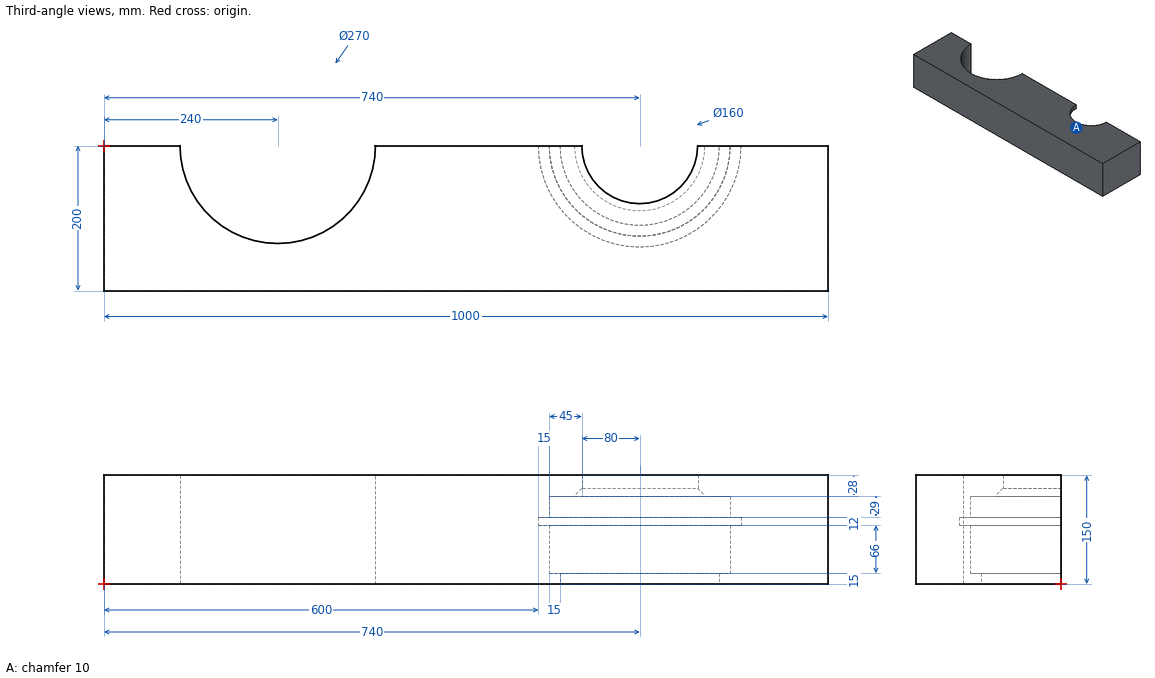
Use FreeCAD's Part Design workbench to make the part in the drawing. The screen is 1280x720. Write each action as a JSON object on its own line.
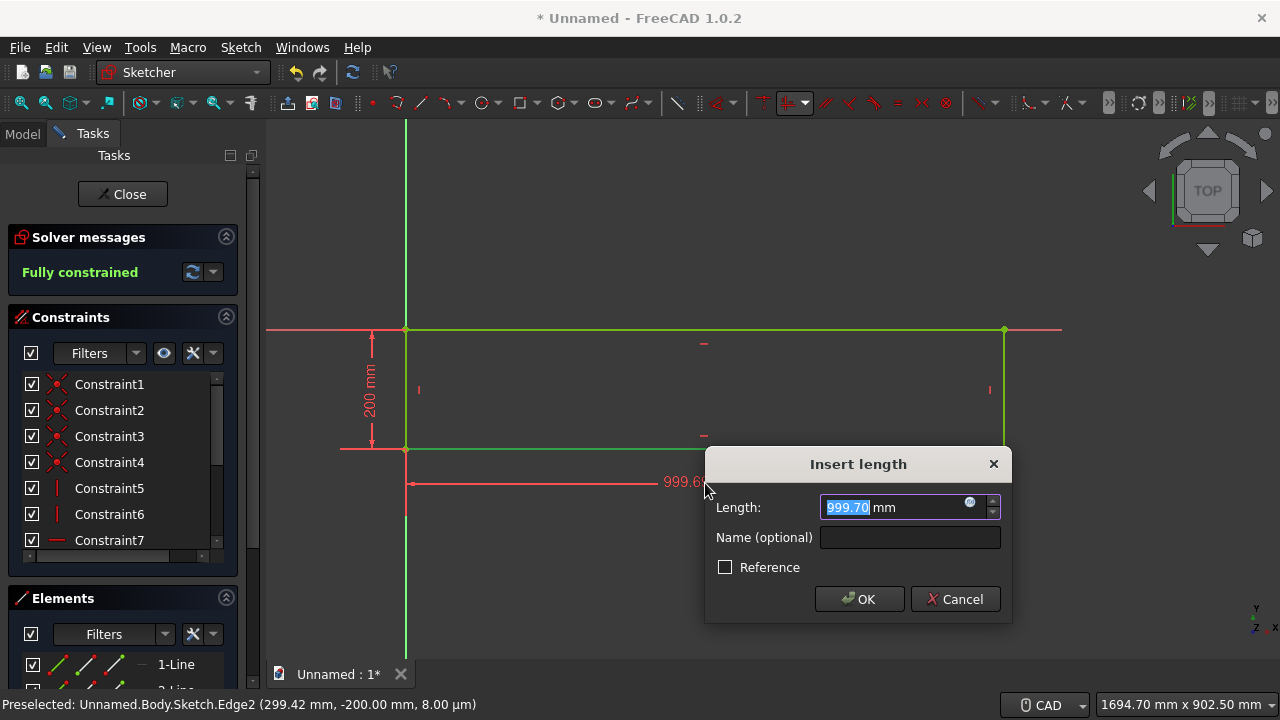
{"action": "type", "text": "1000"}
{"action": "key", "text": "Return"}
{"action": "key", "text": "Escape"}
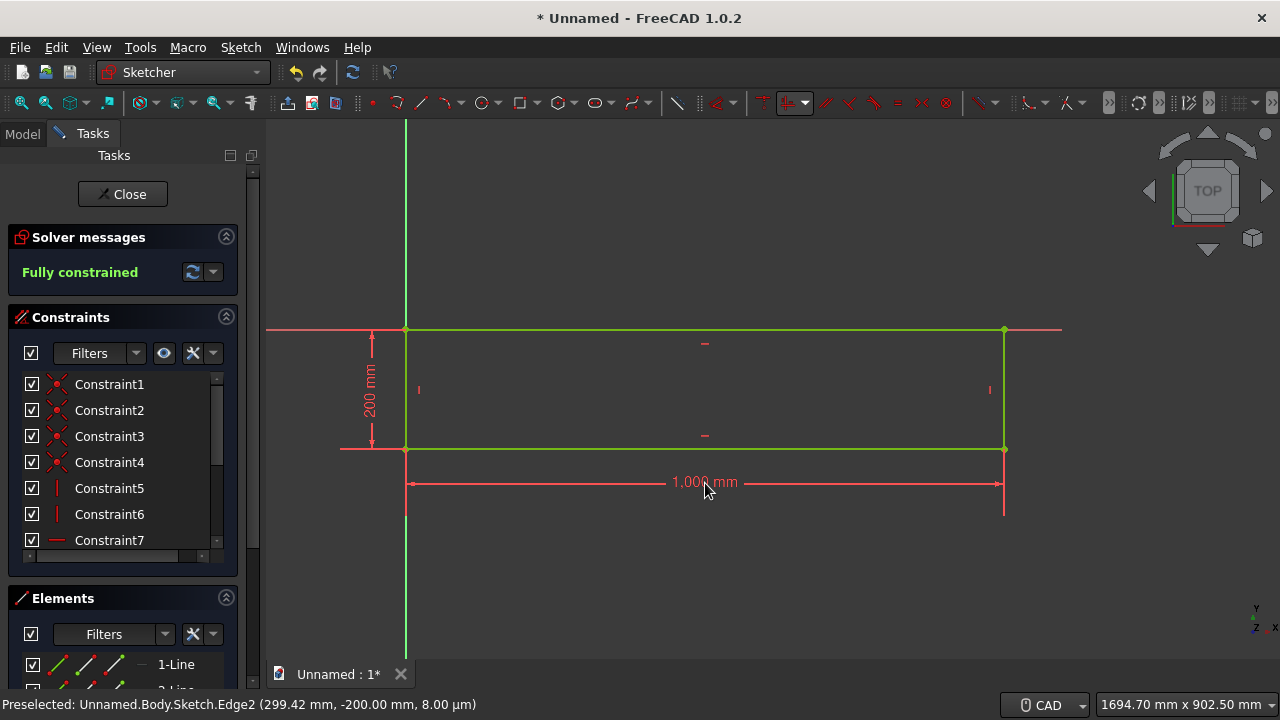
{"action": "left_click", "coordinate": [123, 194]}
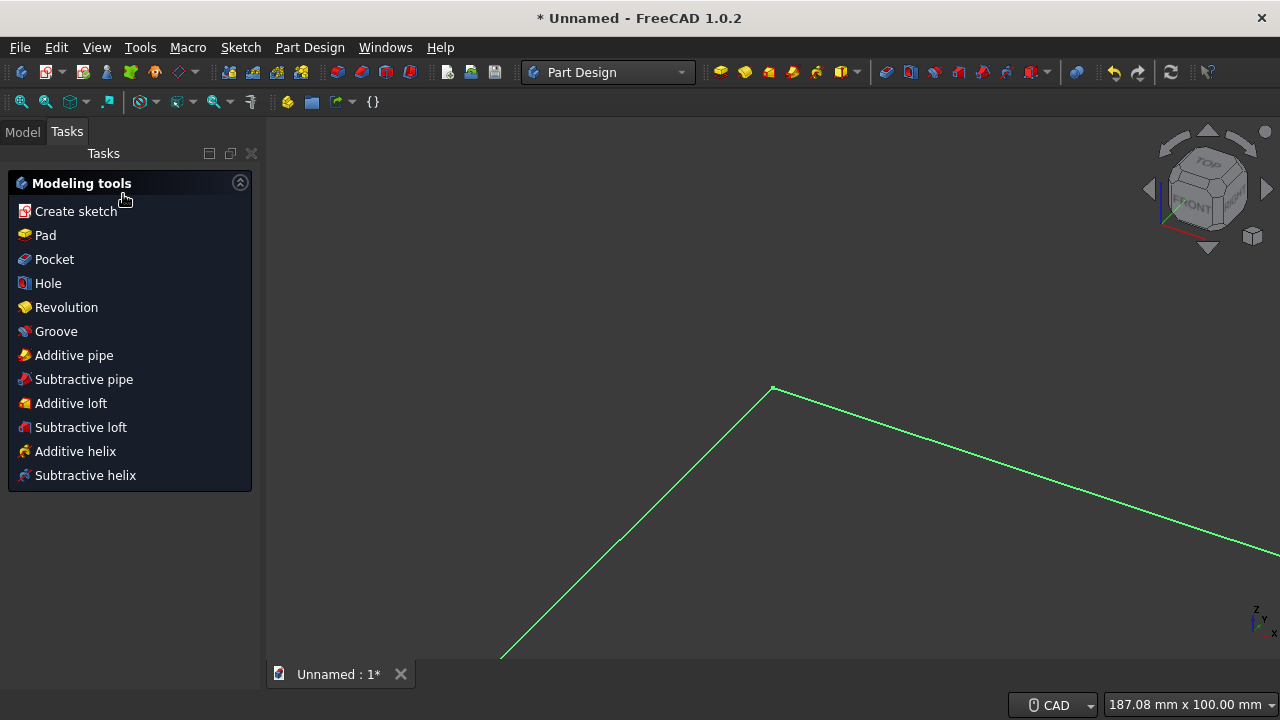
{"action": "left_click", "coordinate": [722, 72]}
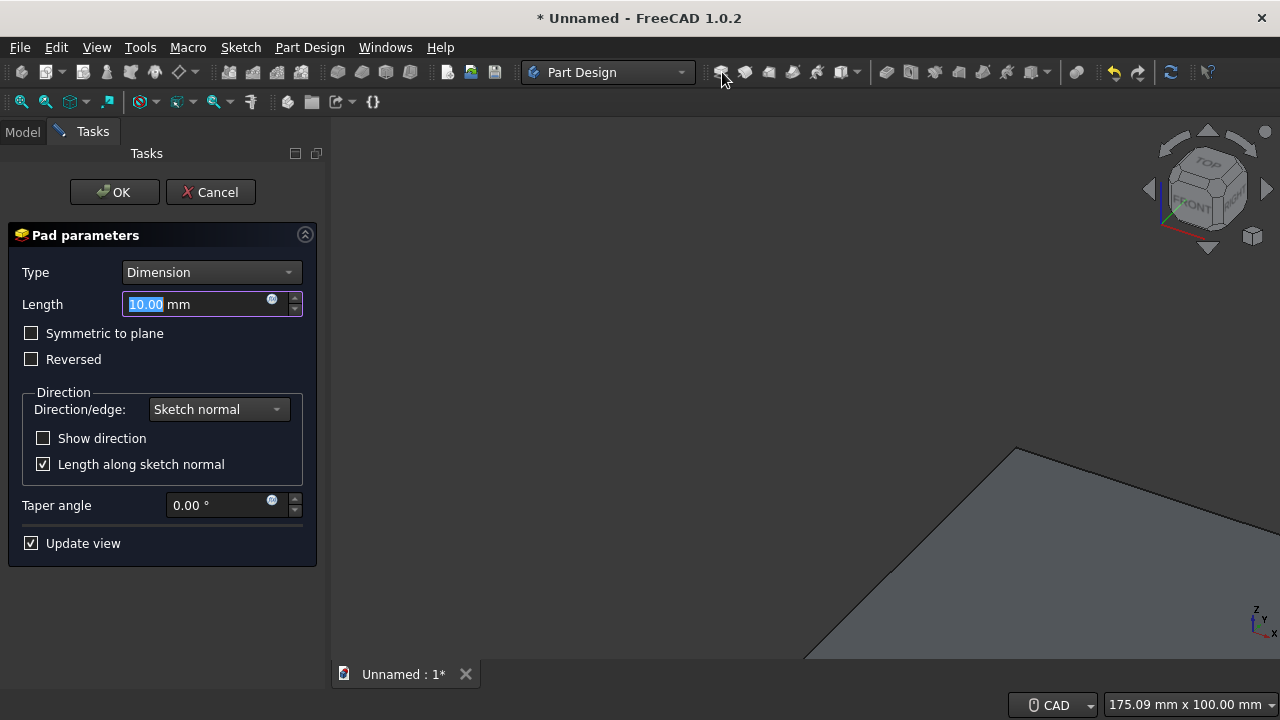
{"action": "type", "text": "150"}
{"action": "key", "text": "Tab"}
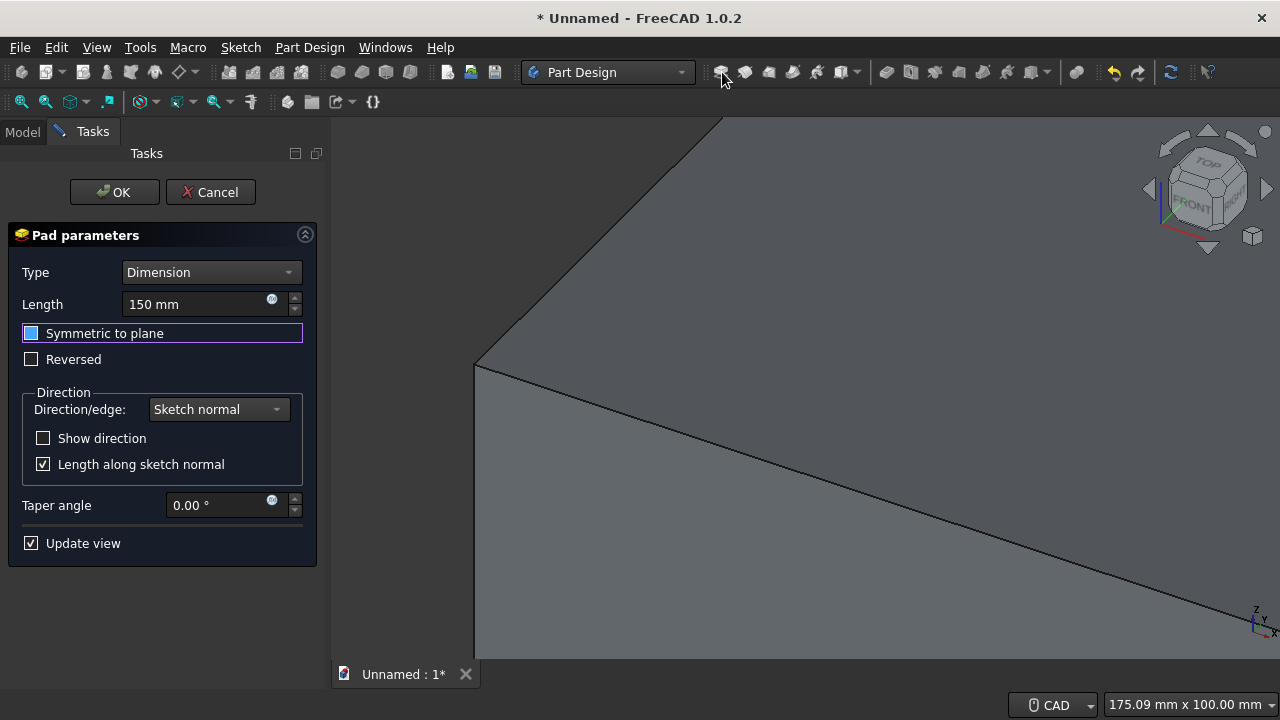
{"action": "left_click", "coordinate": [115, 192]}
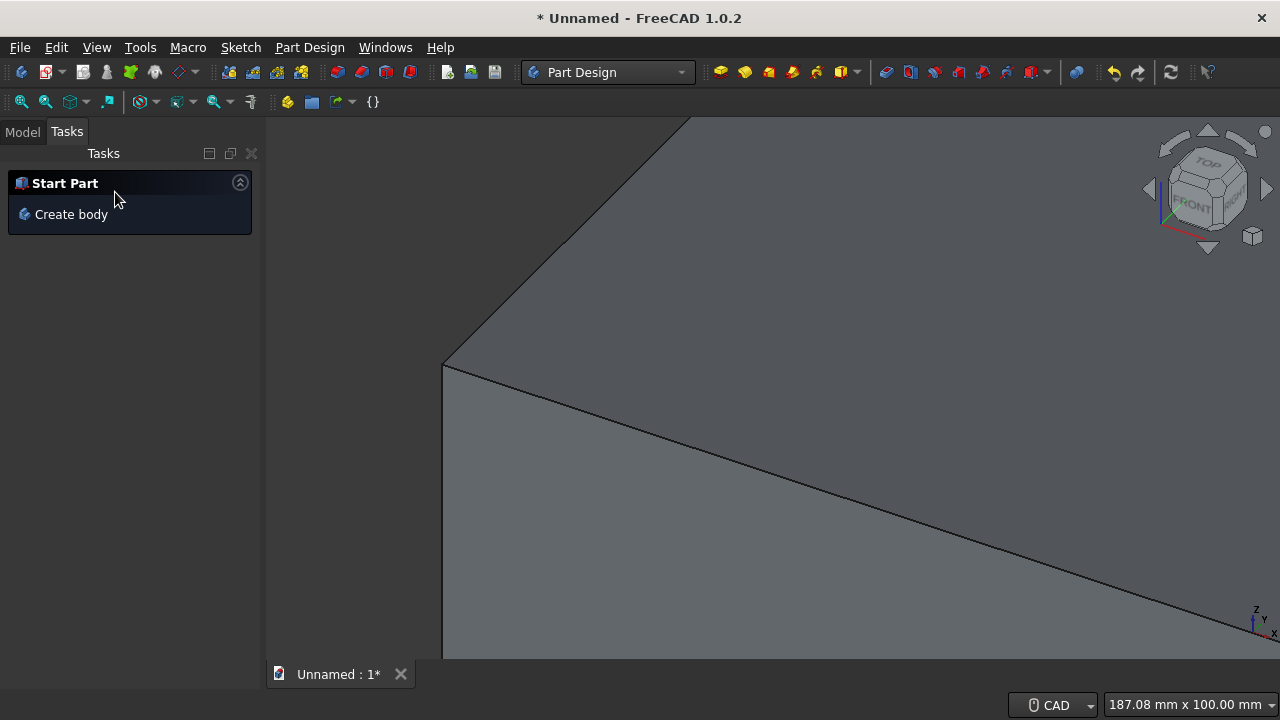
{"action": "left_click", "coordinate": [22, 102]}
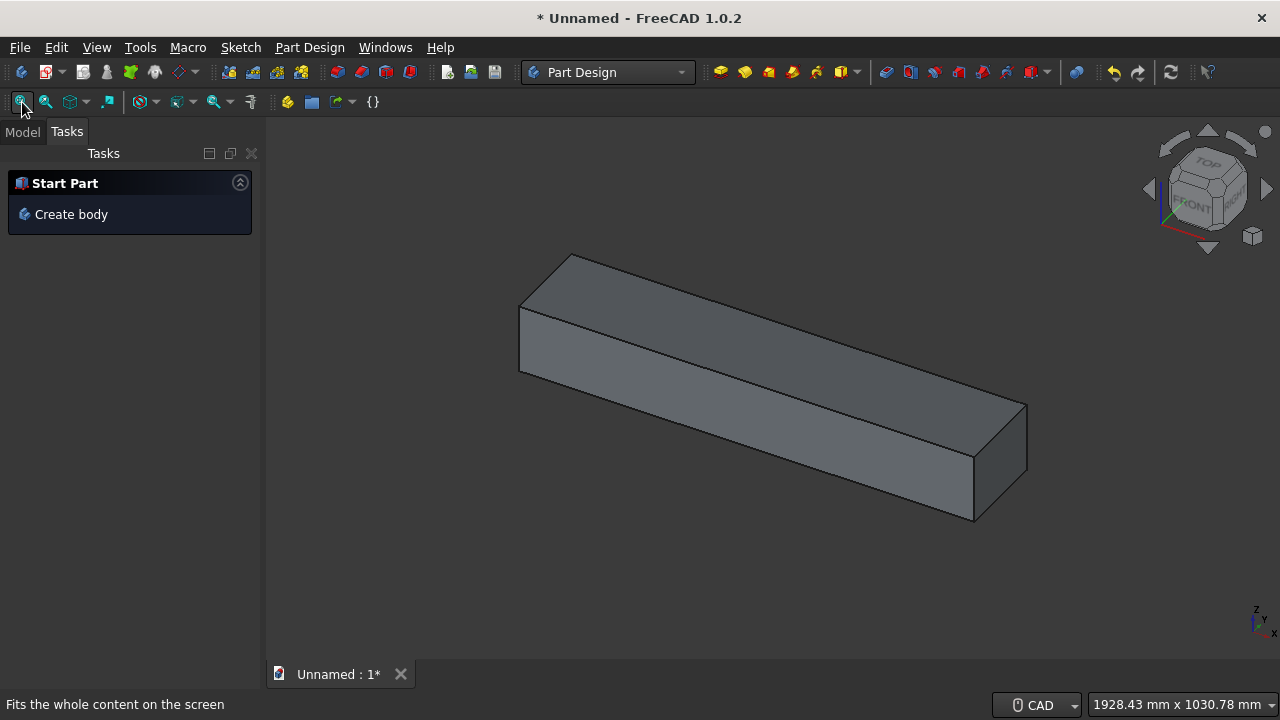
{"action": "left_click", "coordinate": [903, 398]}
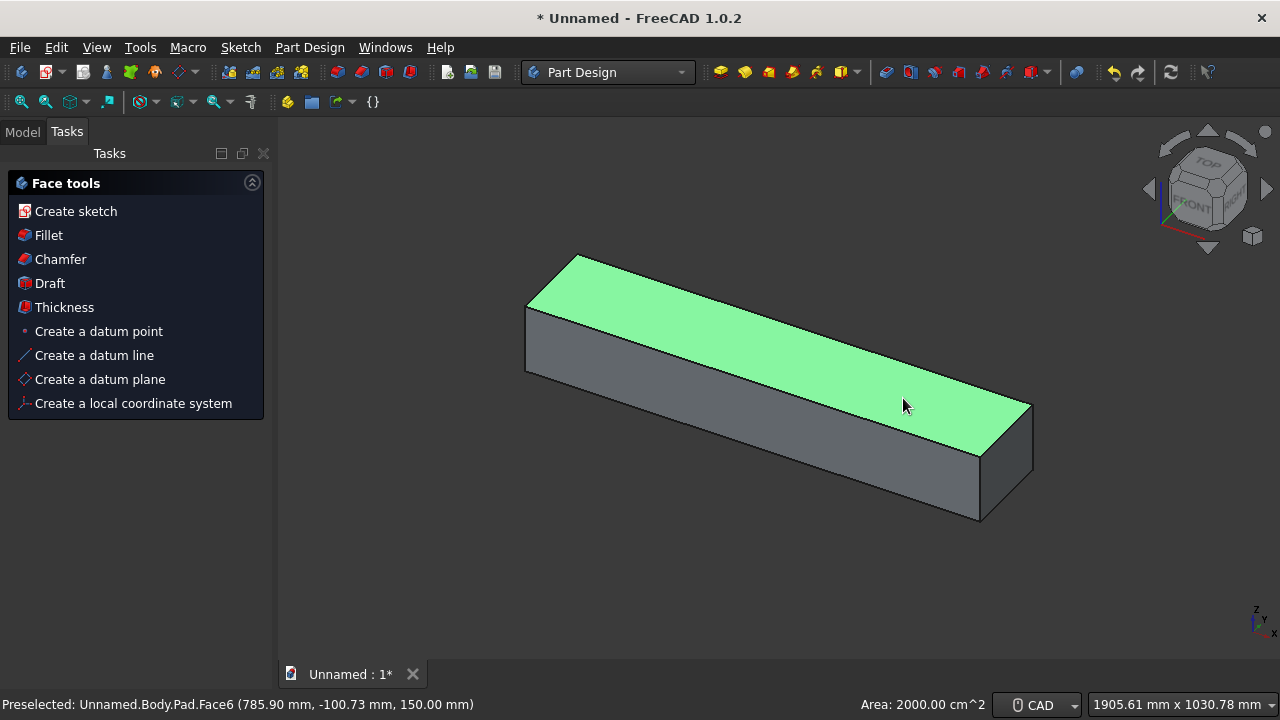
{"action": "left_click", "coordinate": [46, 72]}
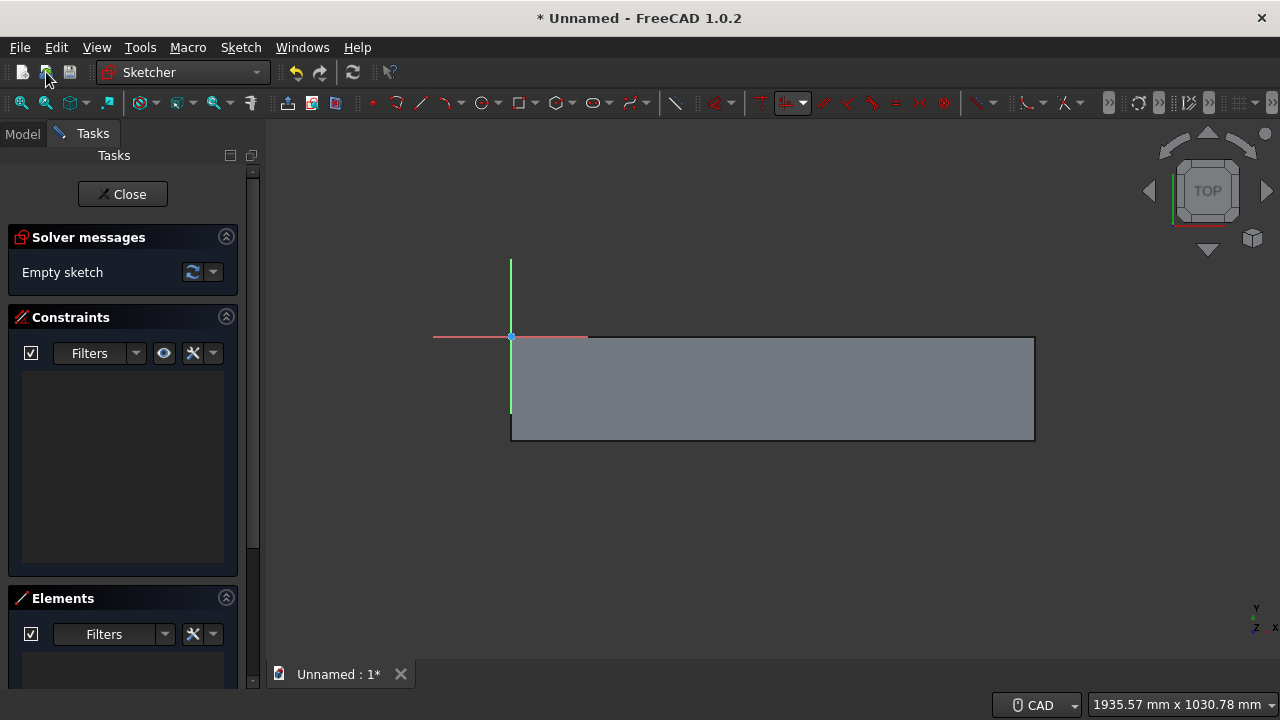
{"action": "left_click", "coordinate": [482, 104]}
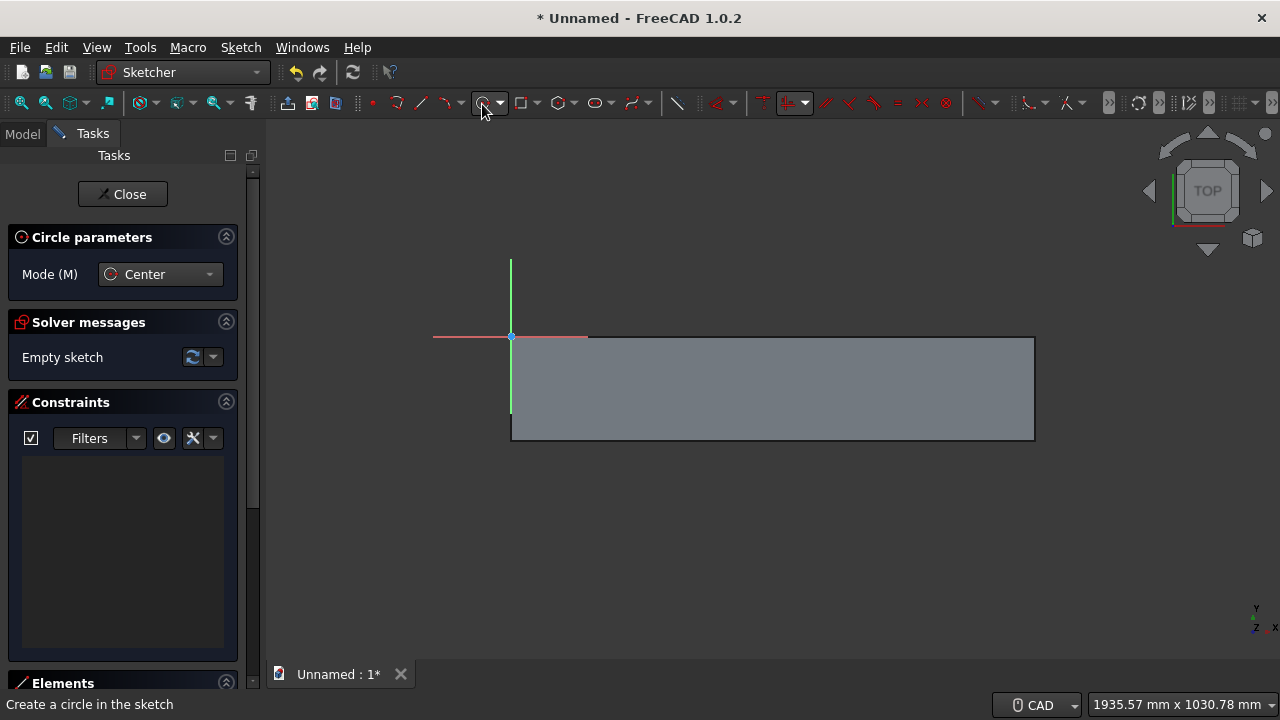
{"action": "left_click", "coordinate": [637, 337]}
{"action": "left_click", "coordinate": [687, 287]}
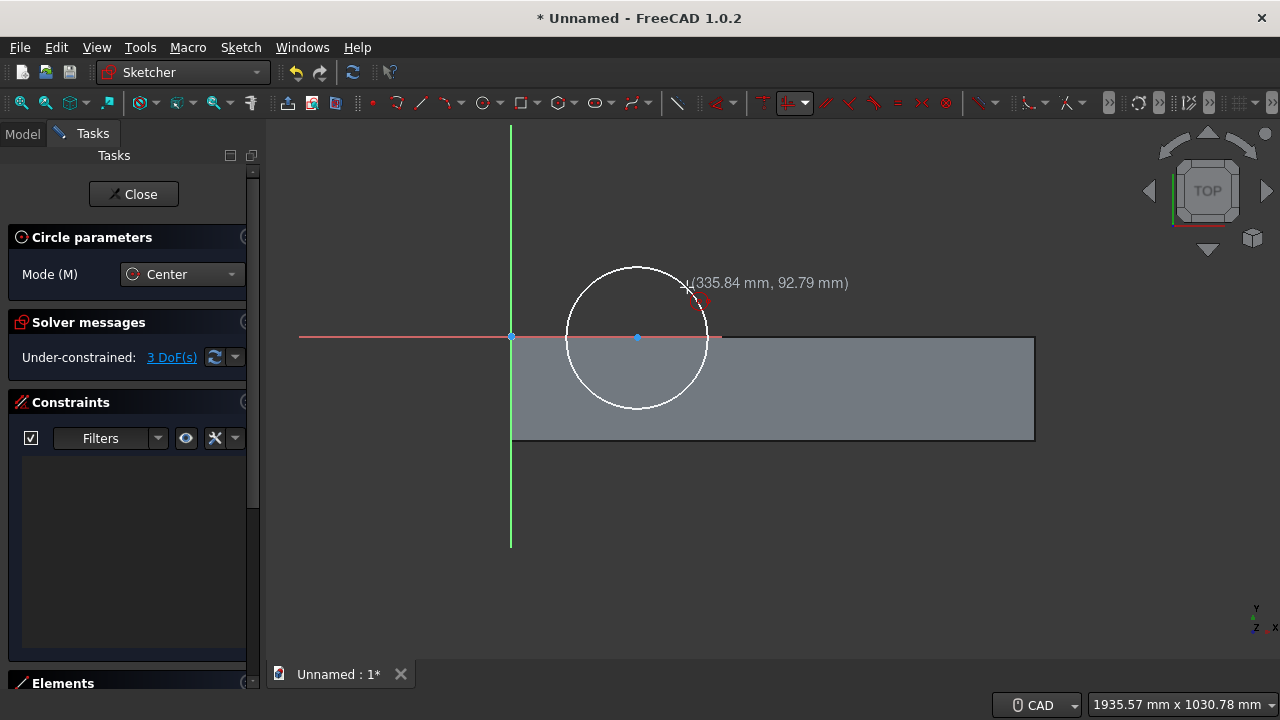
{"action": "left_click", "coordinate": [899, 337]}
{"action": "left_click", "coordinate": [928, 307]}
{"action": "key", "text": "Escape"}